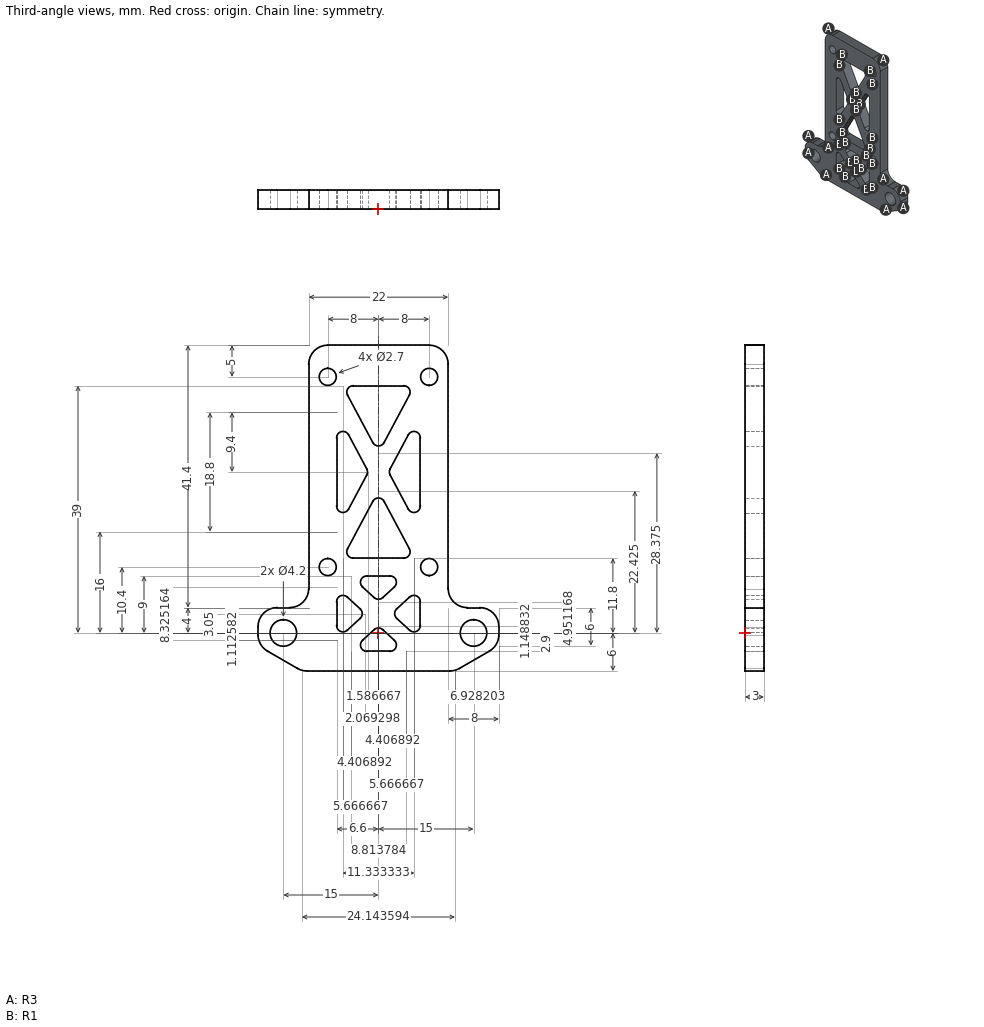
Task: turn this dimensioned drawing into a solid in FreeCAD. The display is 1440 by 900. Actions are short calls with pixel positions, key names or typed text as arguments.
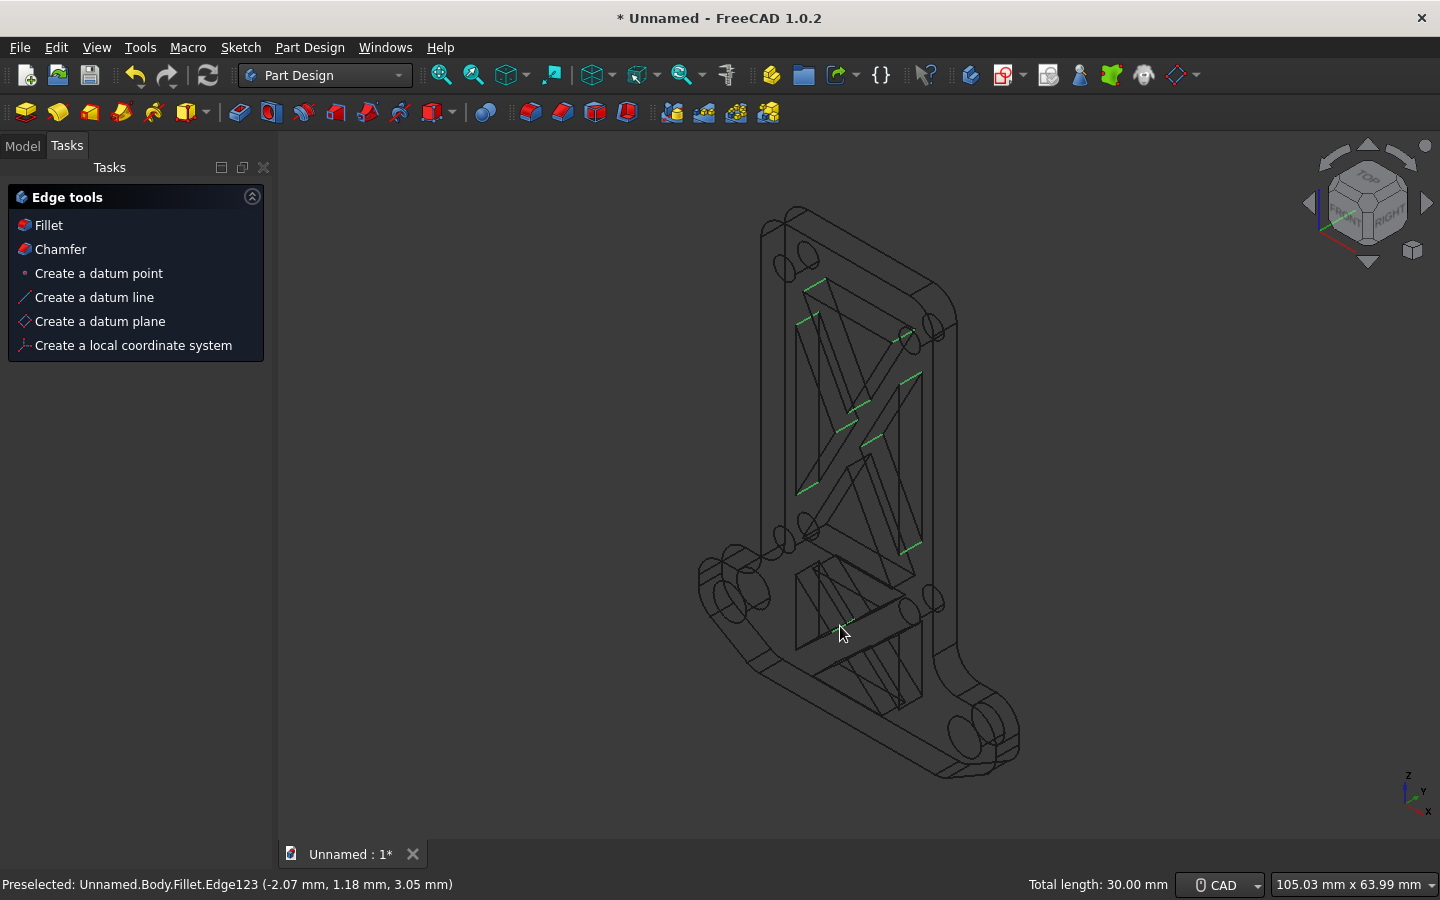
click(805, 568, ctrl)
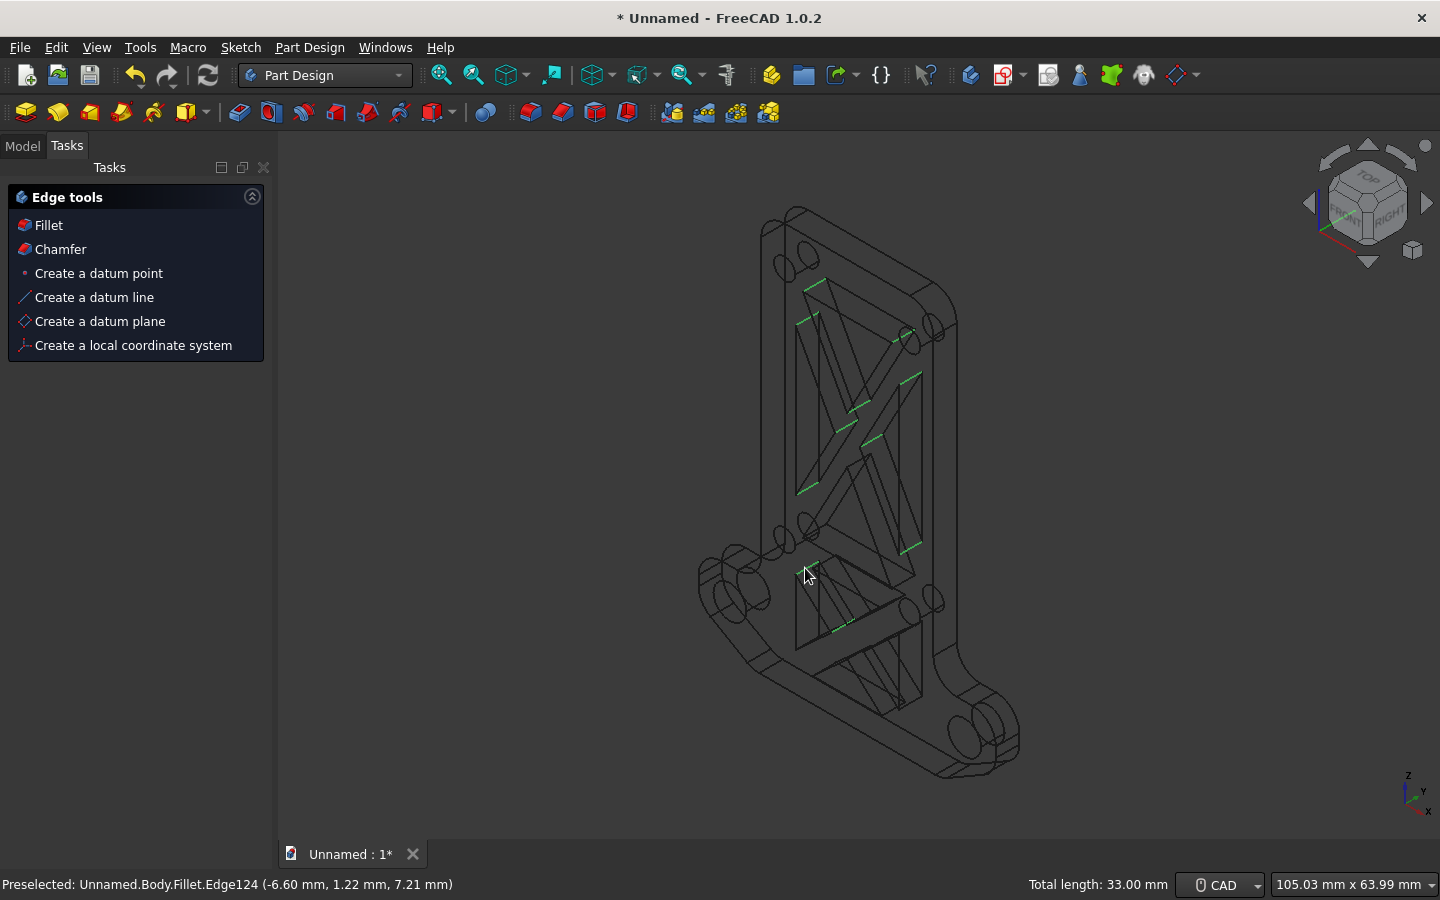
click(815, 530, ctrl)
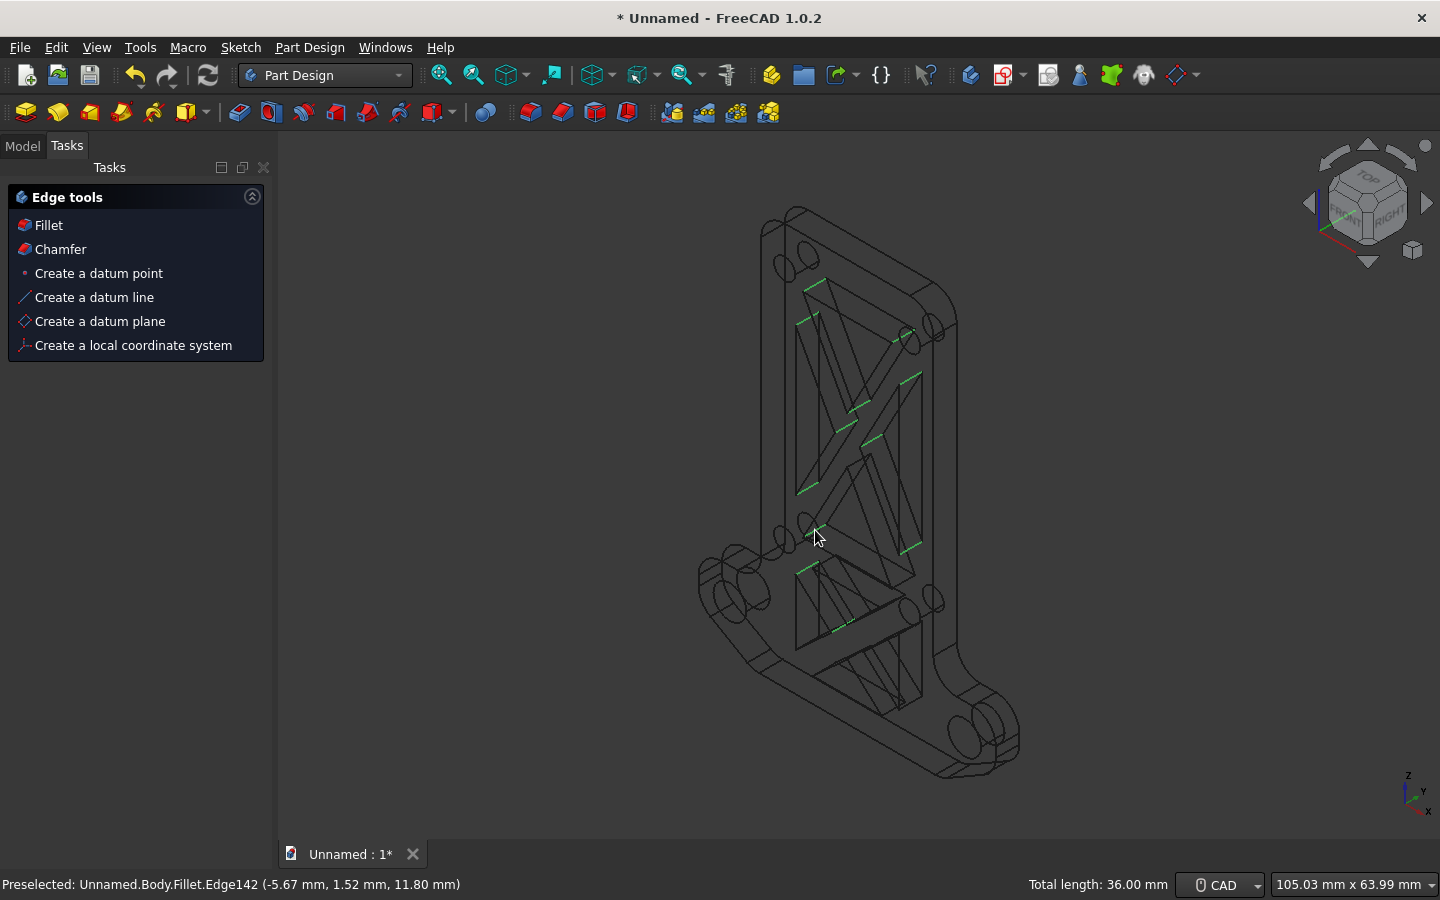
click(903, 581, ctrl)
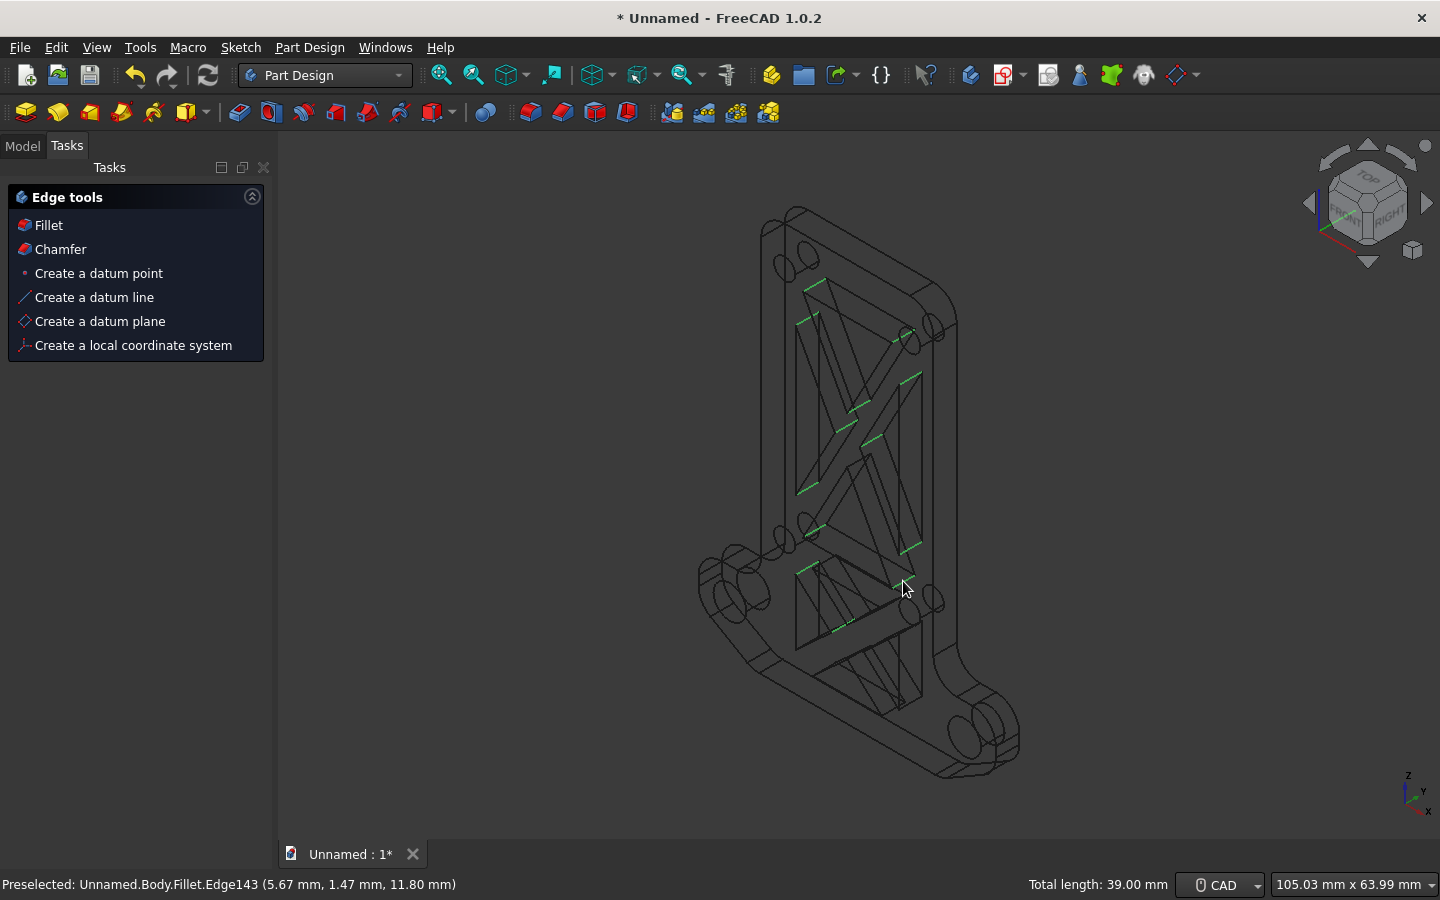
click(857, 461, ctrl)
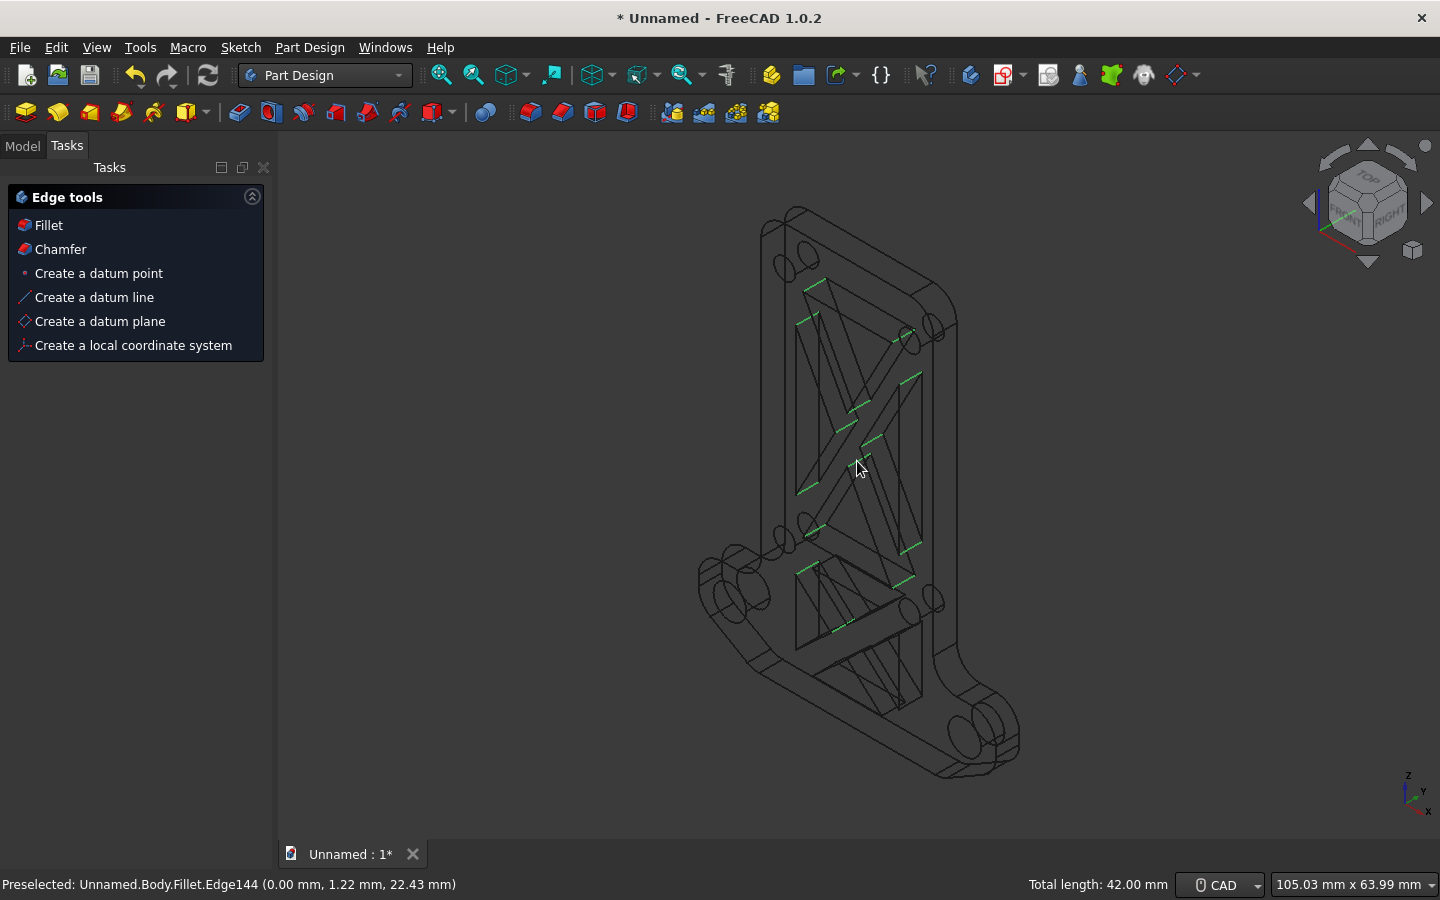
click(893, 601, ctrl)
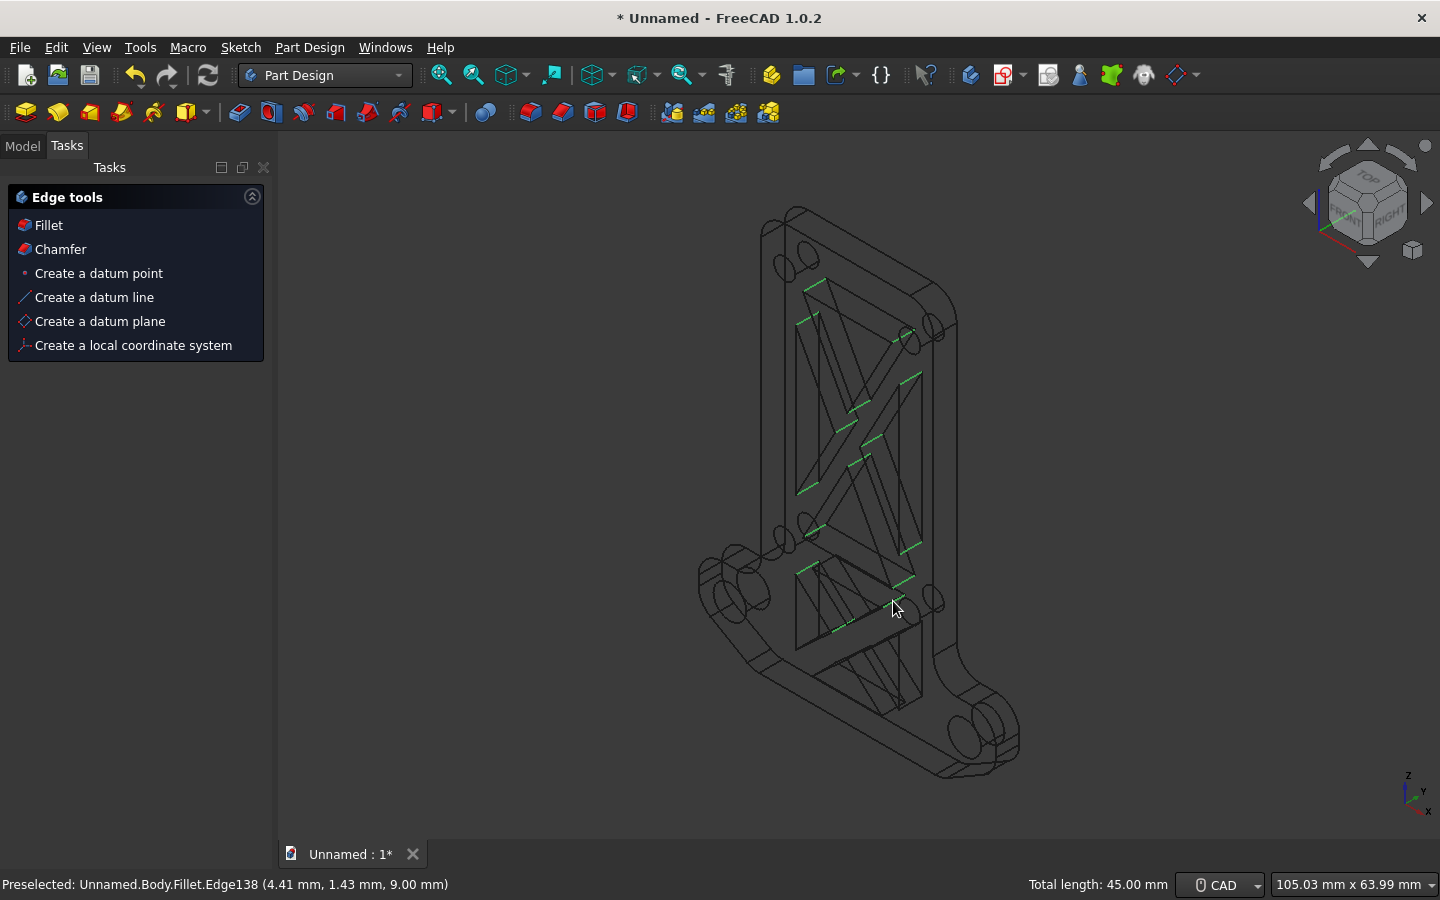
click(825, 561, ctrl)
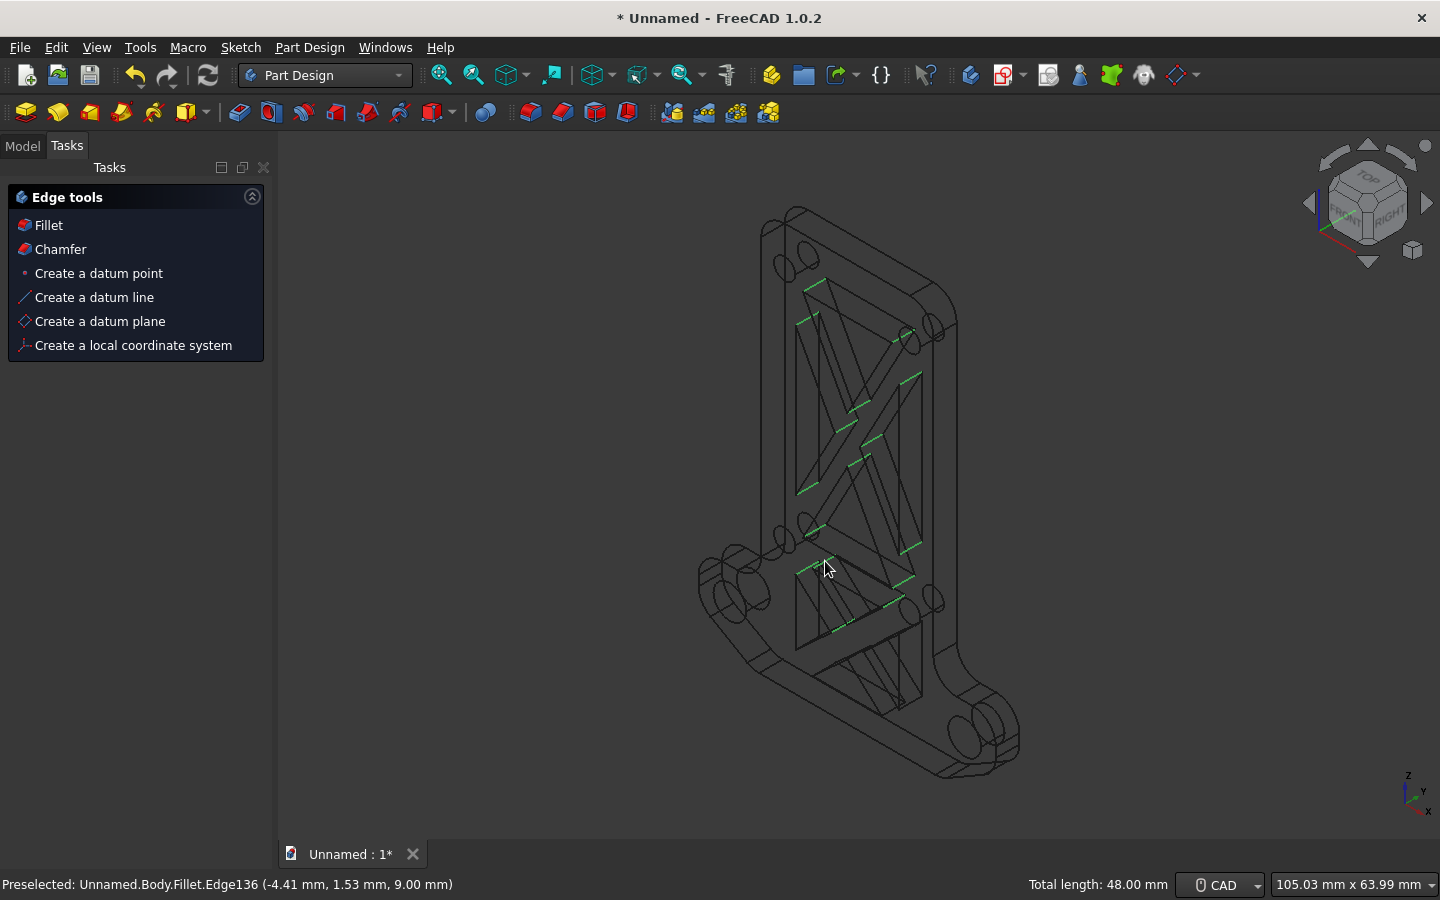
click(891, 709, ctrl)